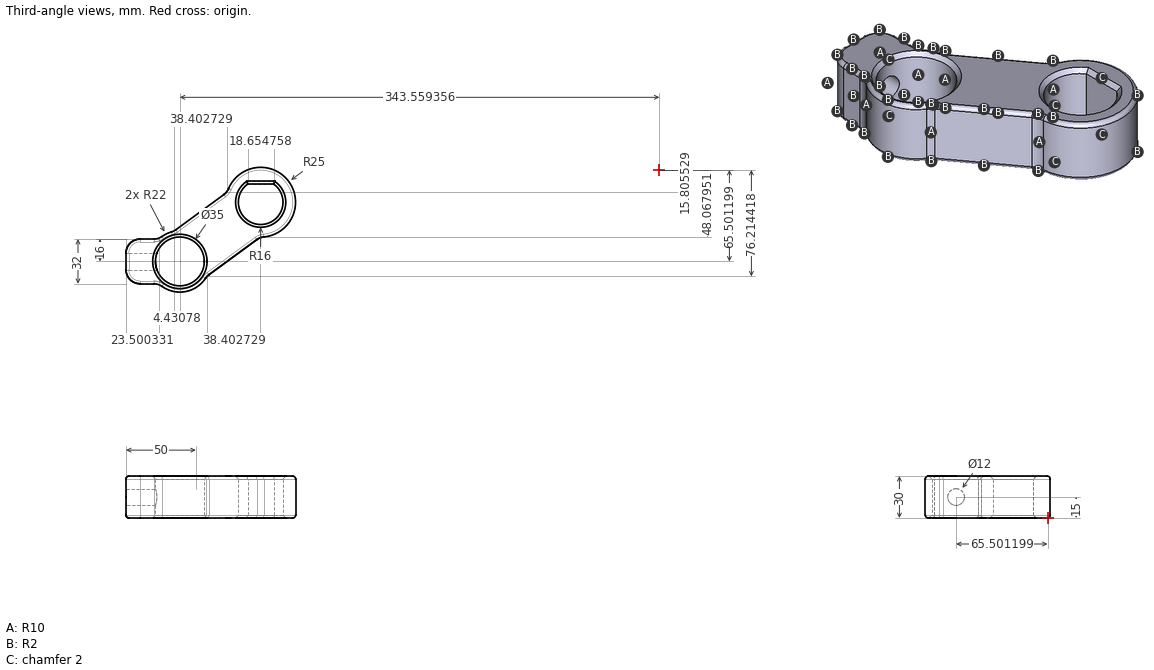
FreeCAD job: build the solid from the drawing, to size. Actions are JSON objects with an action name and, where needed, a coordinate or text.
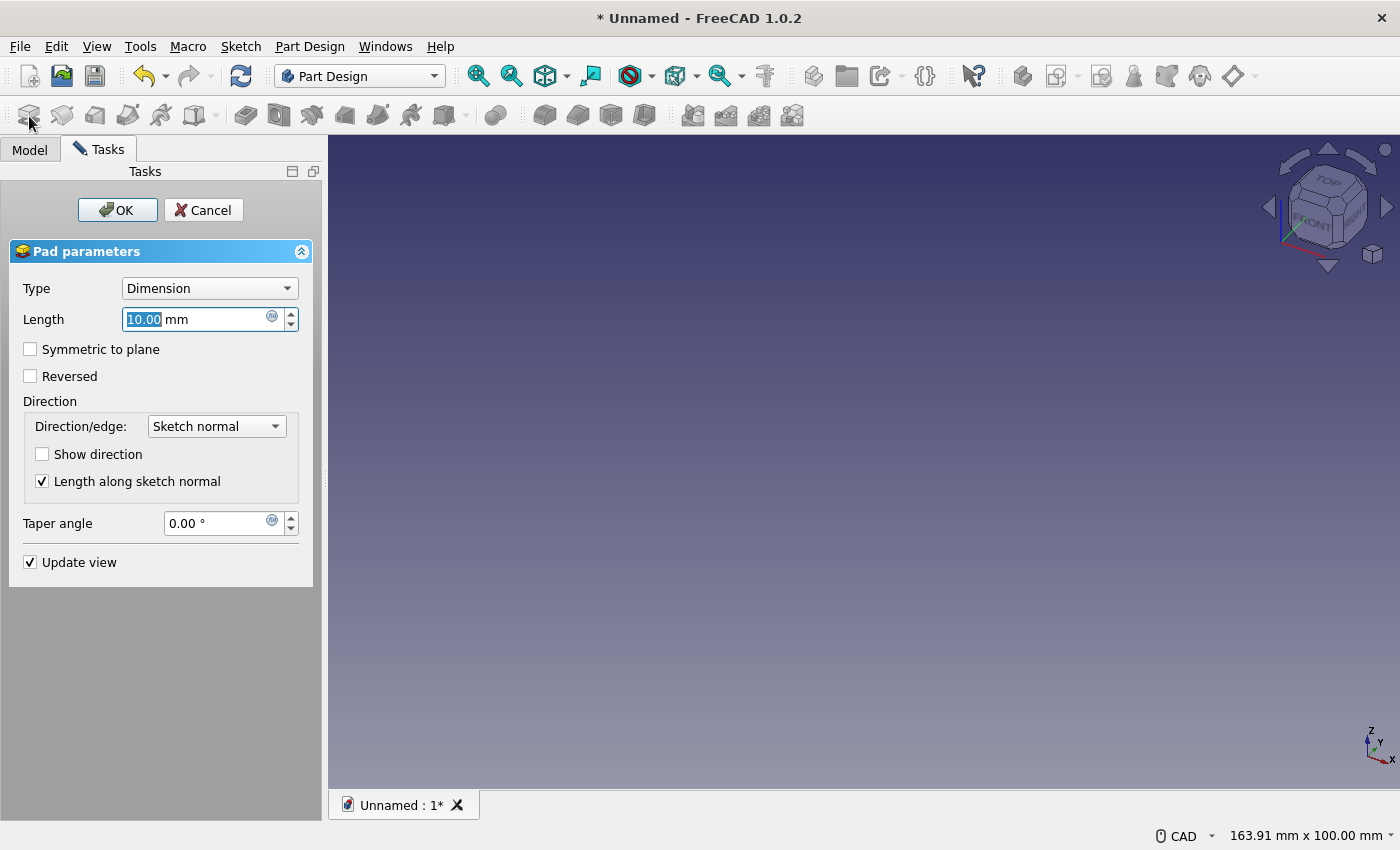
{"action": "type", "text": "30"}
{"action": "key", "text": "Tab"}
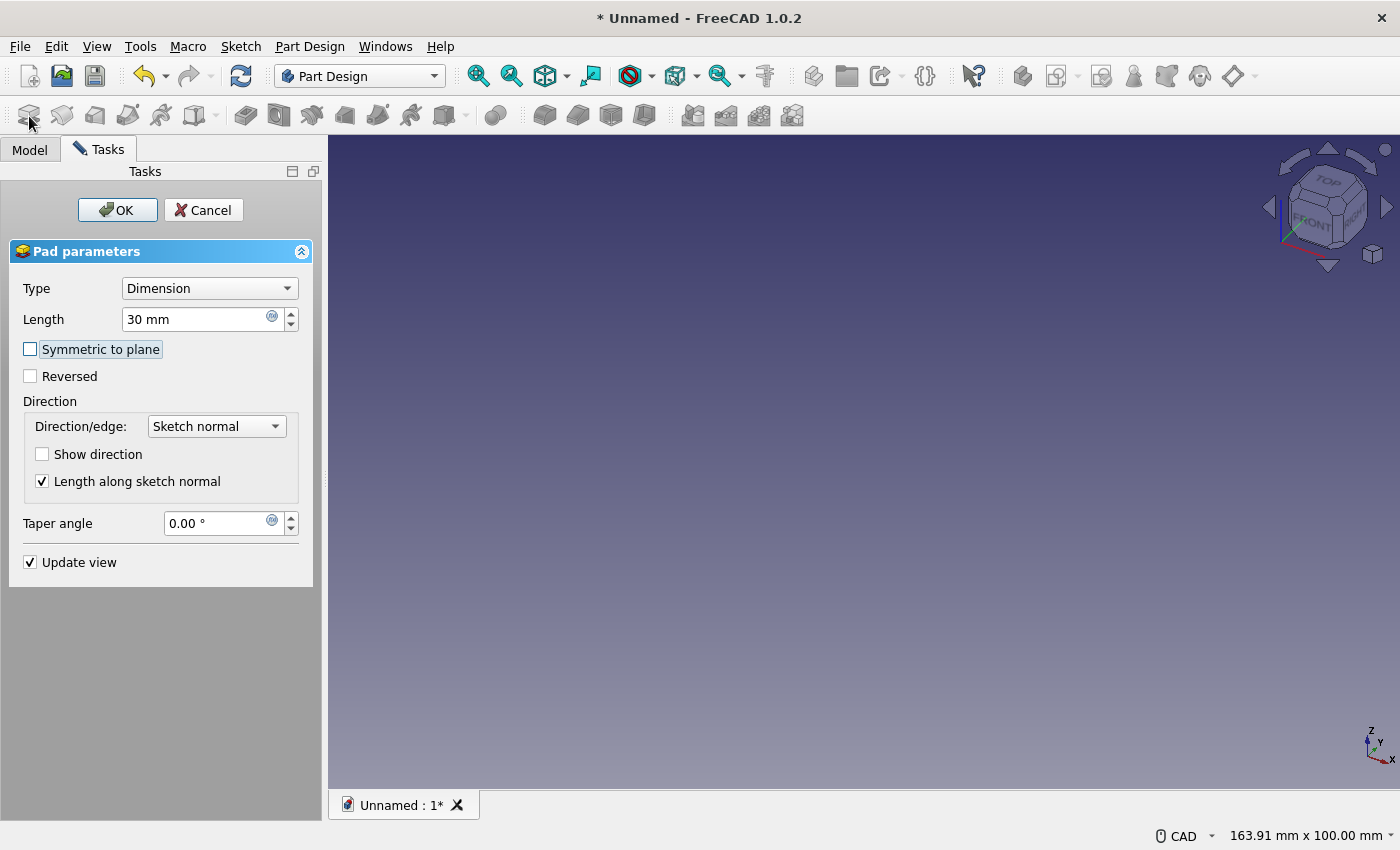
{"action": "left_click", "coordinate": [118, 210]}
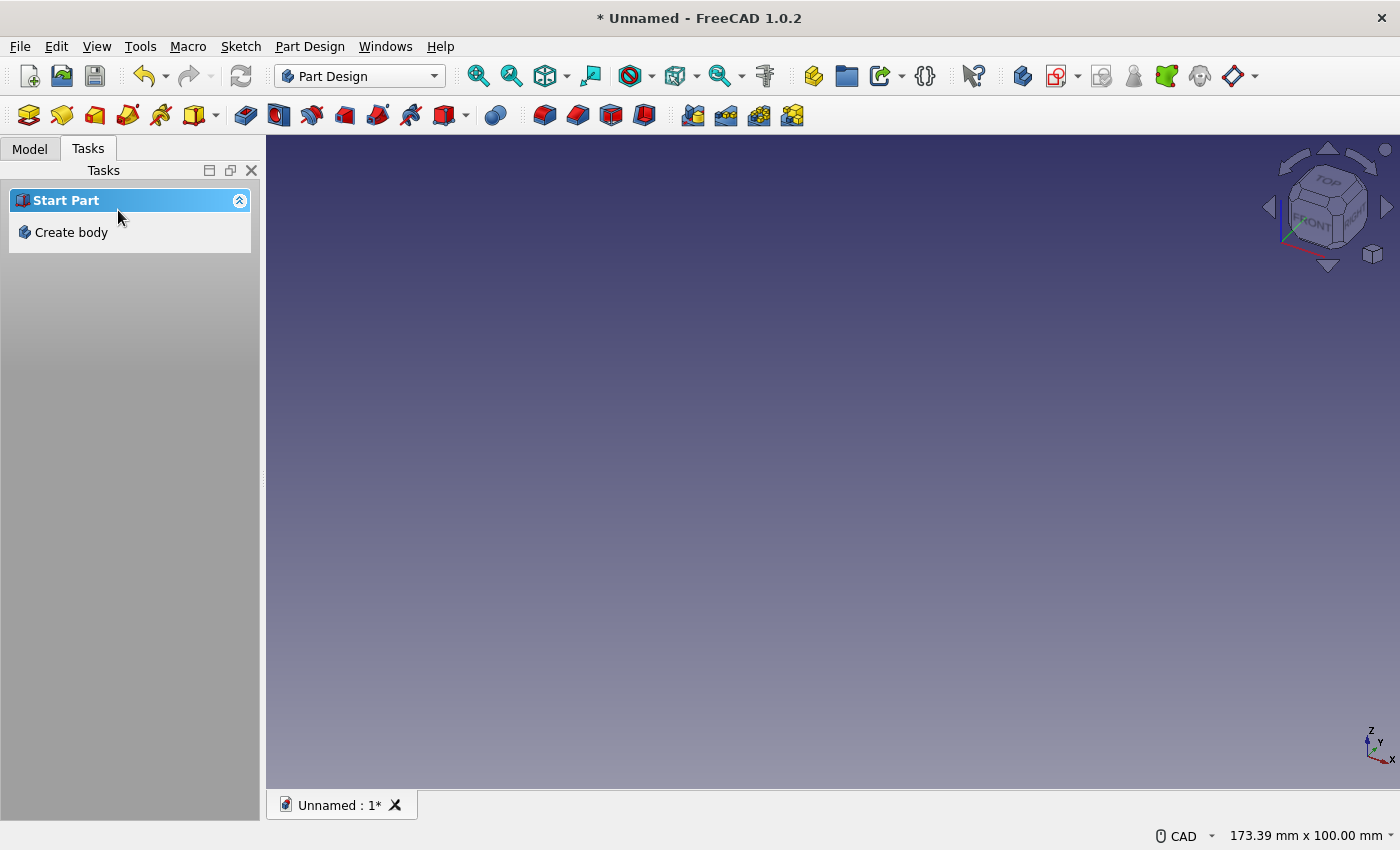
{"action": "left_click", "coordinate": [479, 76]}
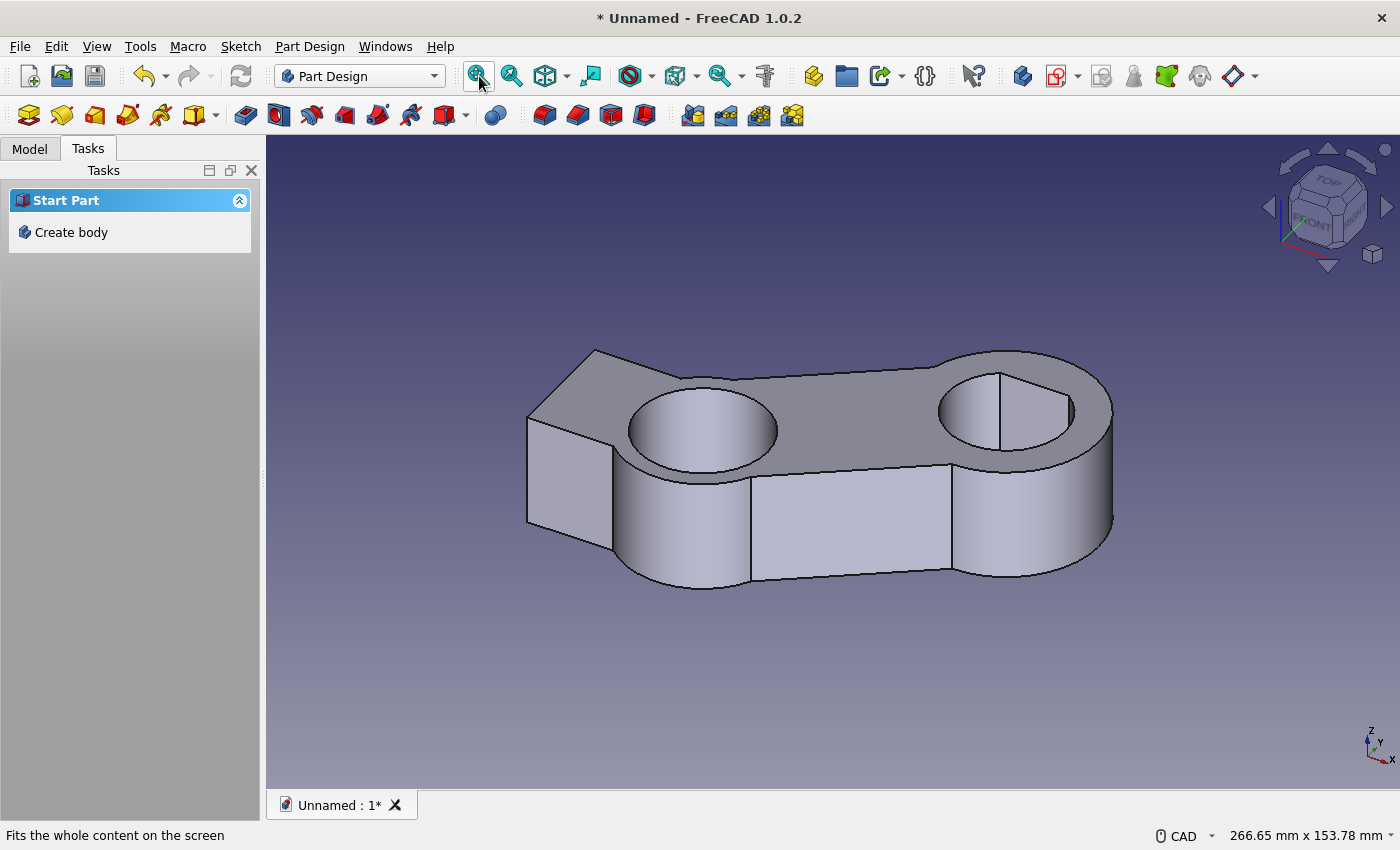
{"action": "key", "text": "0"}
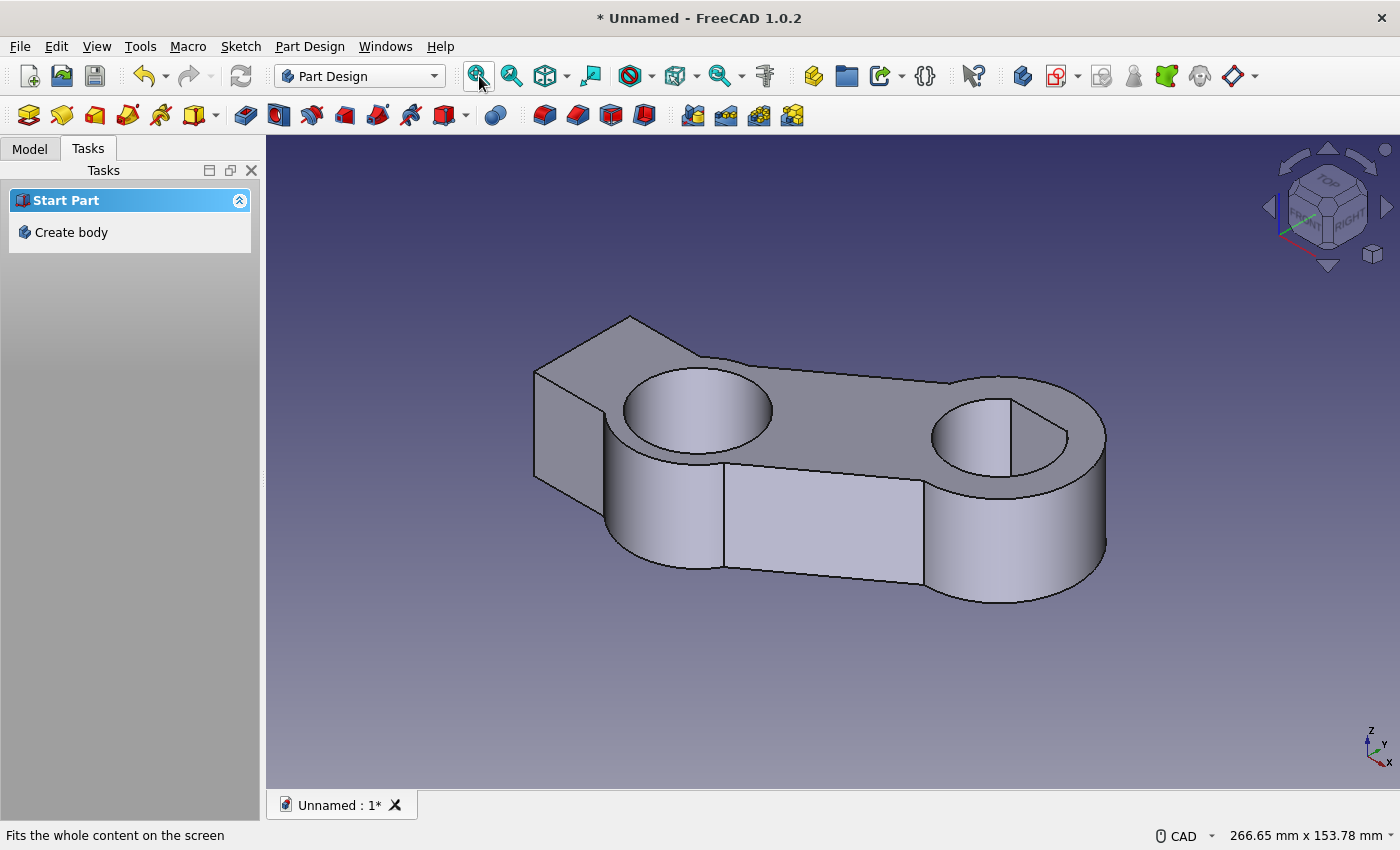
{"action": "key", "text": "2"}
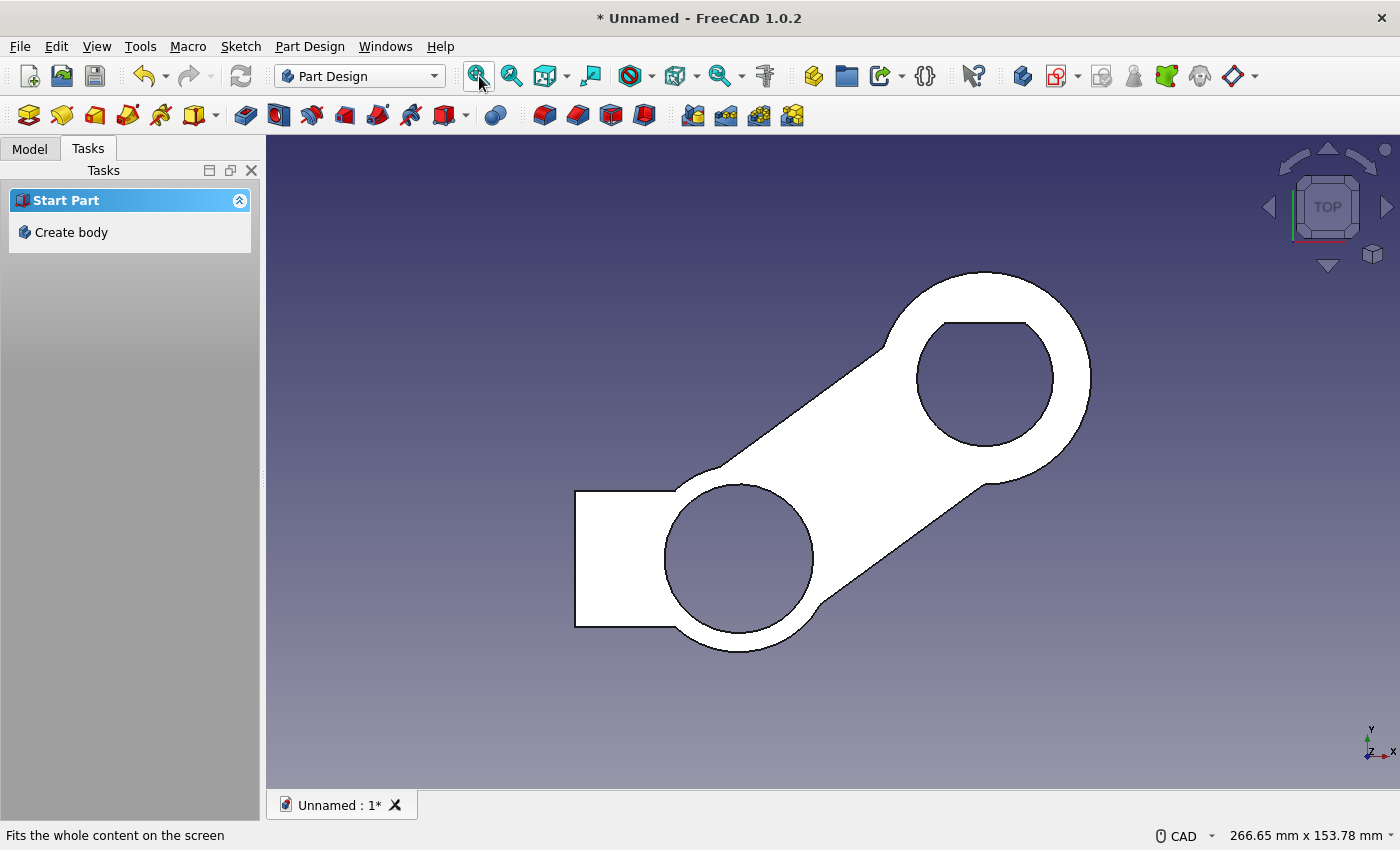
{"action": "key", "text": "1"}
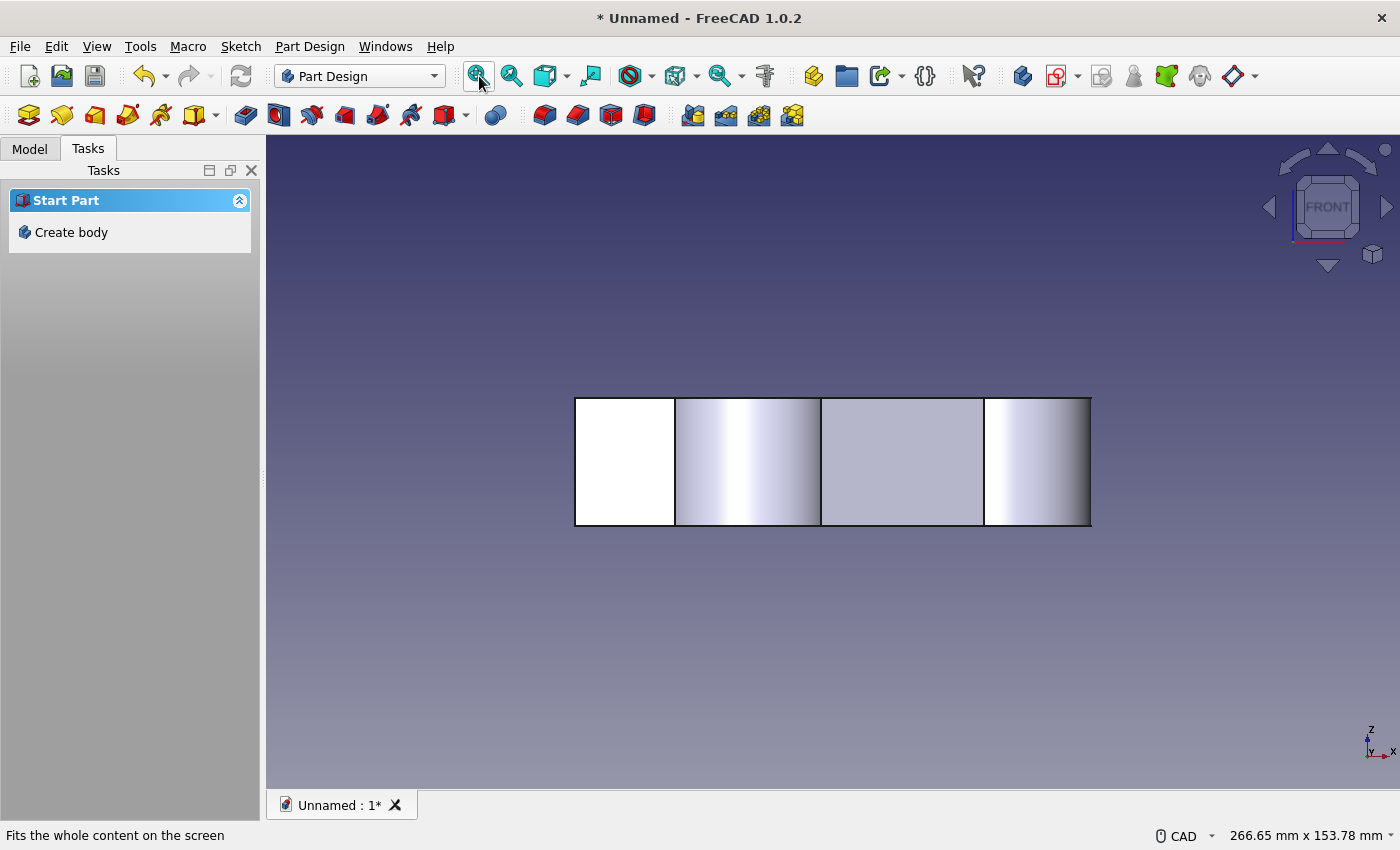
{"action": "left_click", "coordinate": [575, 461]}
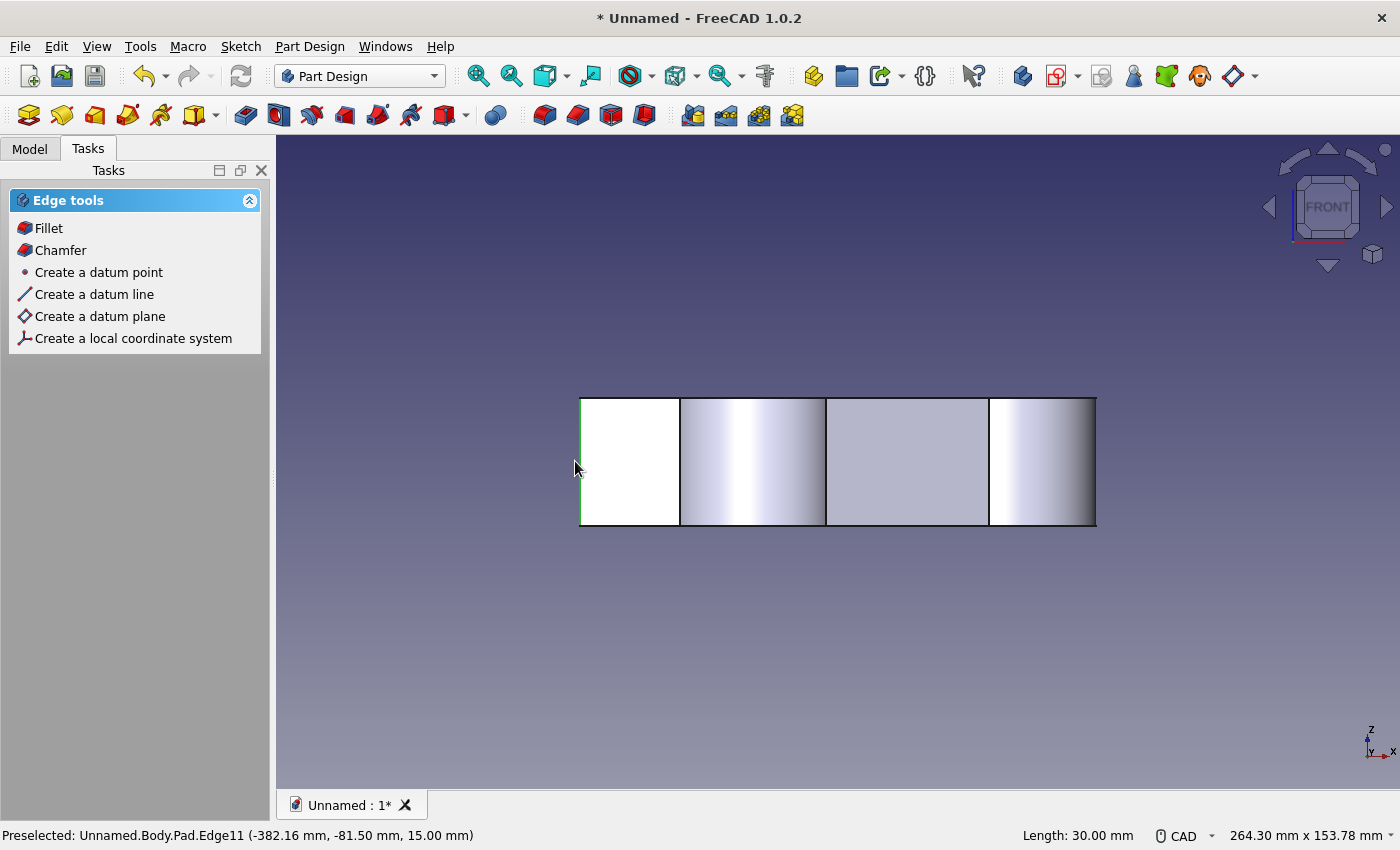
{"action": "key", "text": "3"}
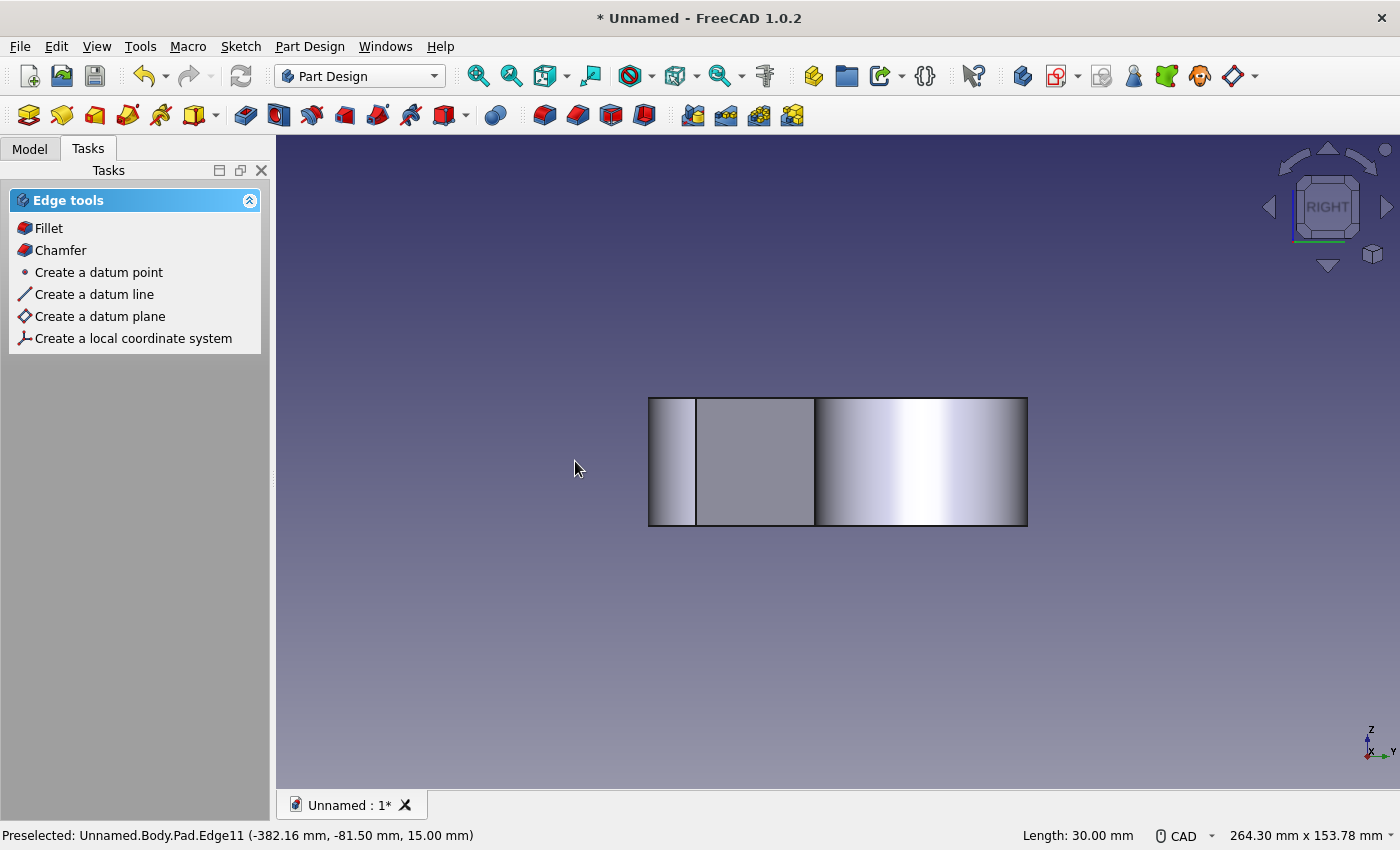
{"action": "key", "text": "v f"}